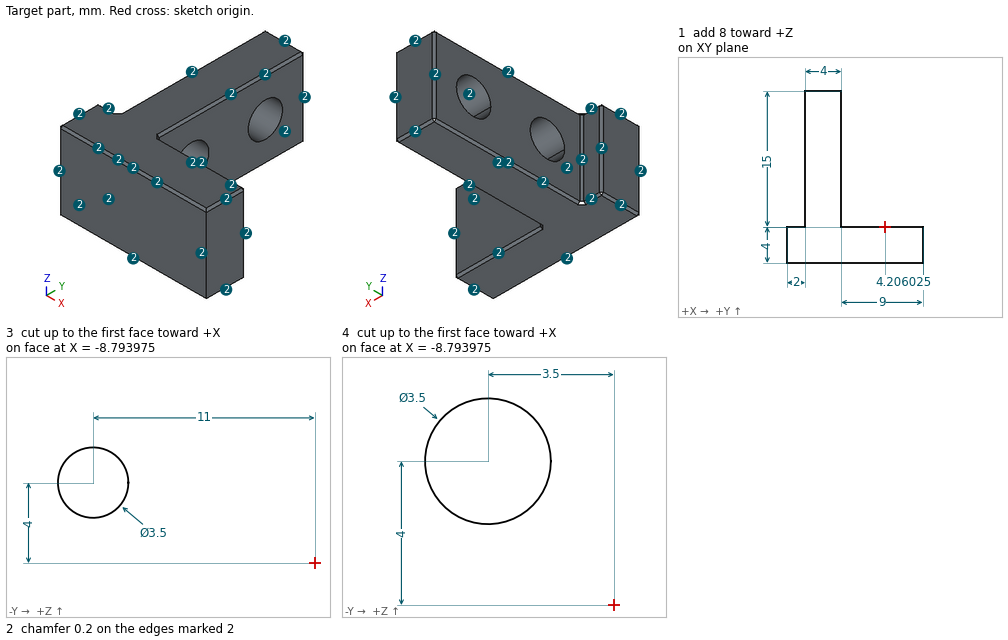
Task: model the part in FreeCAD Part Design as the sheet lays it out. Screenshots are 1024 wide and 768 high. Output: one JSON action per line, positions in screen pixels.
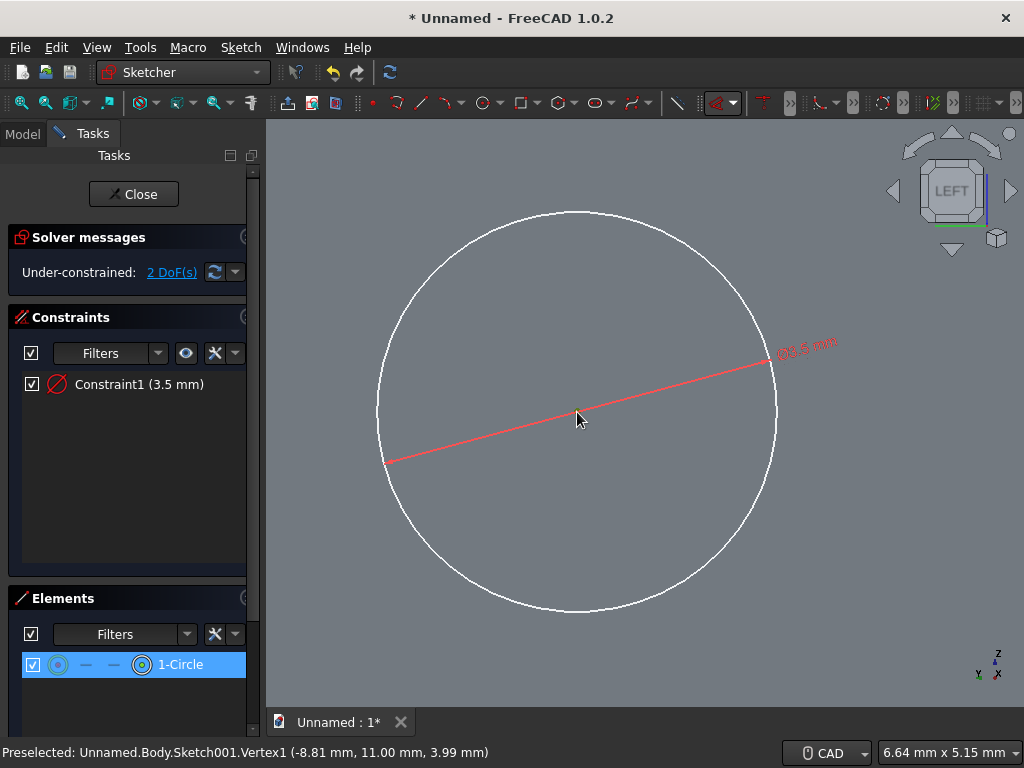
{"action": "left_click", "coordinate": [736, 104]}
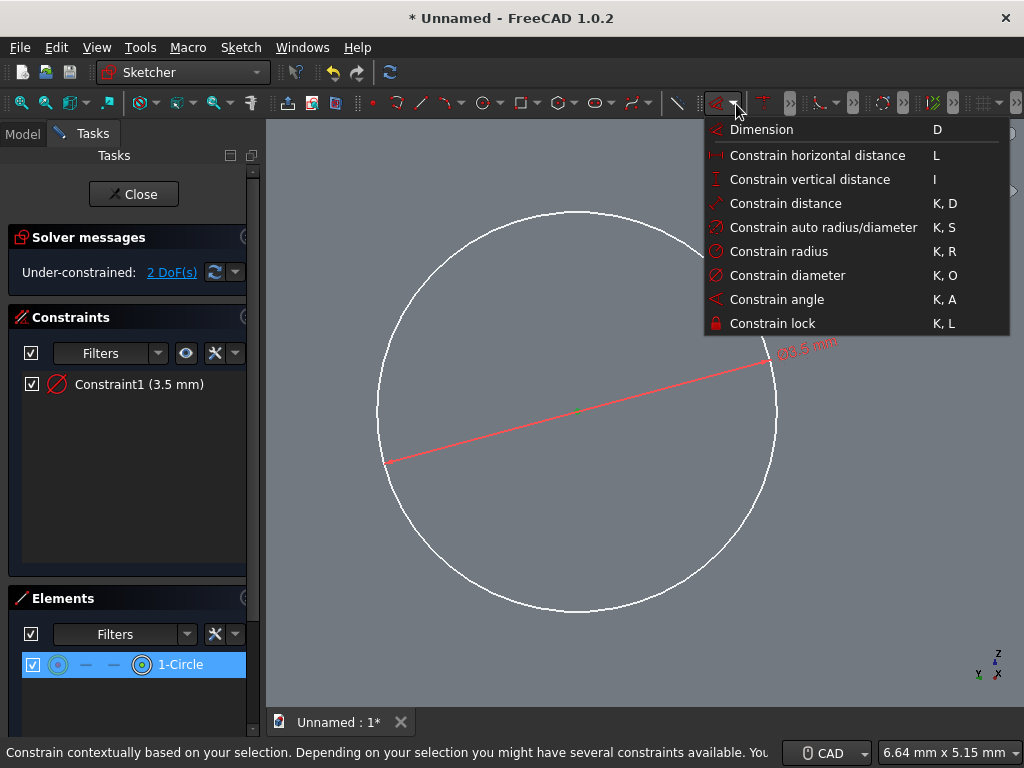
{"action": "left_click", "coordinate": [857, 179]}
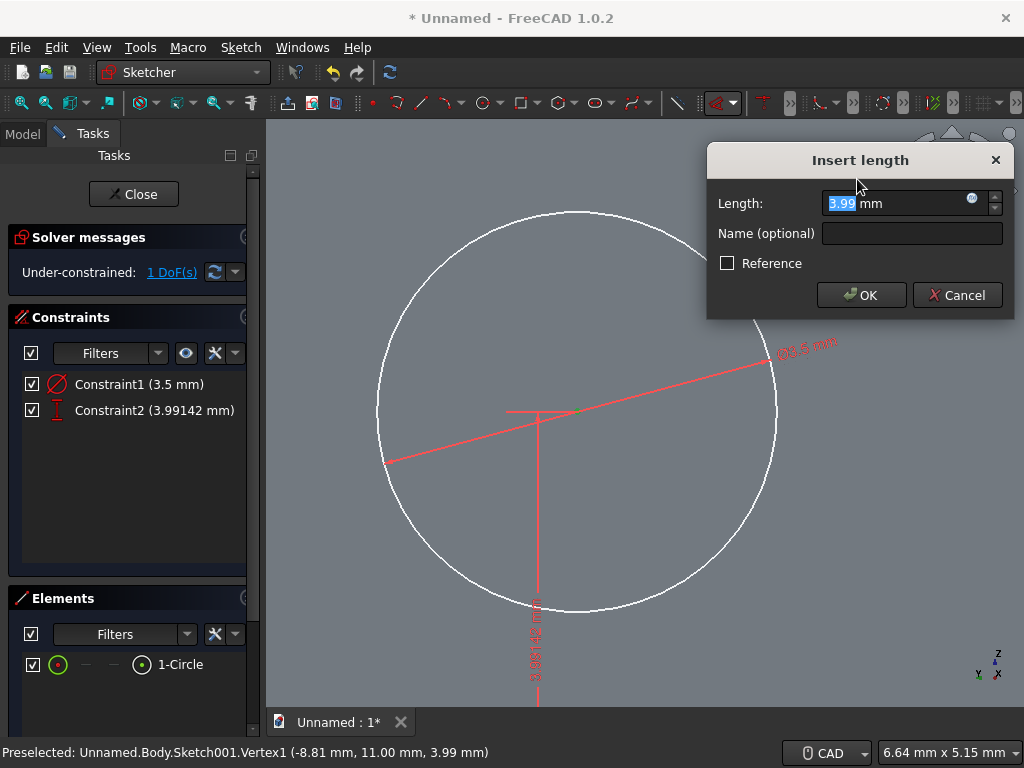
{"action": "type", "text": "4"}
{"action": "key", "text": "Return"}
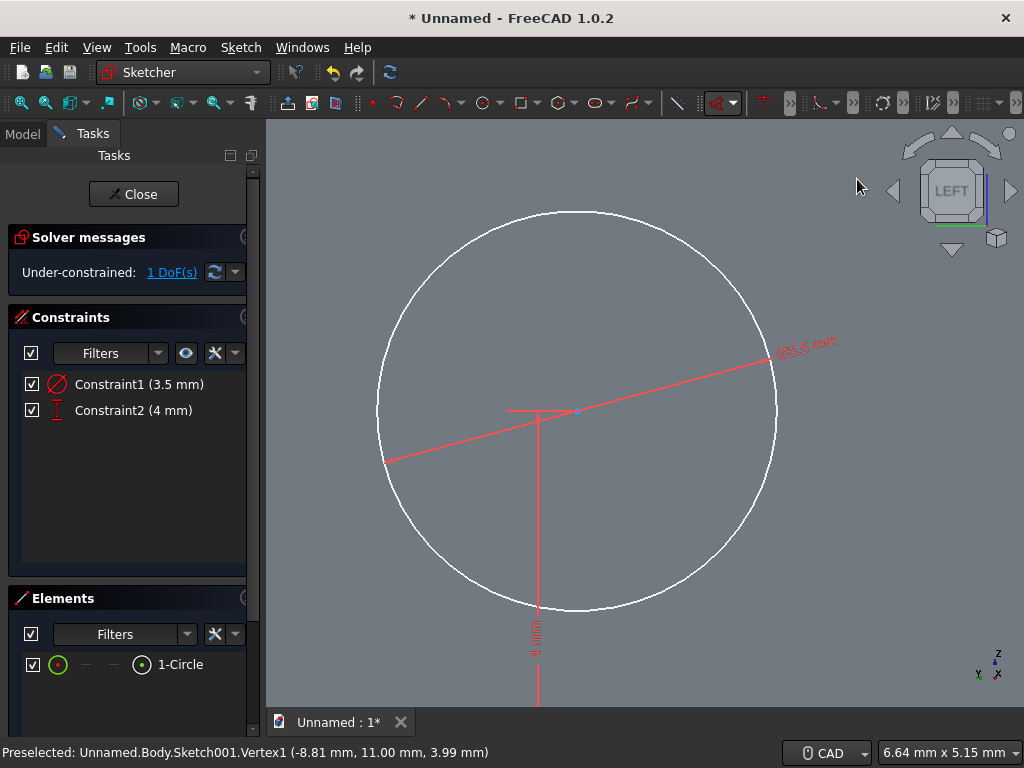
{"action": "left_click", "coordinate": [577, 411]}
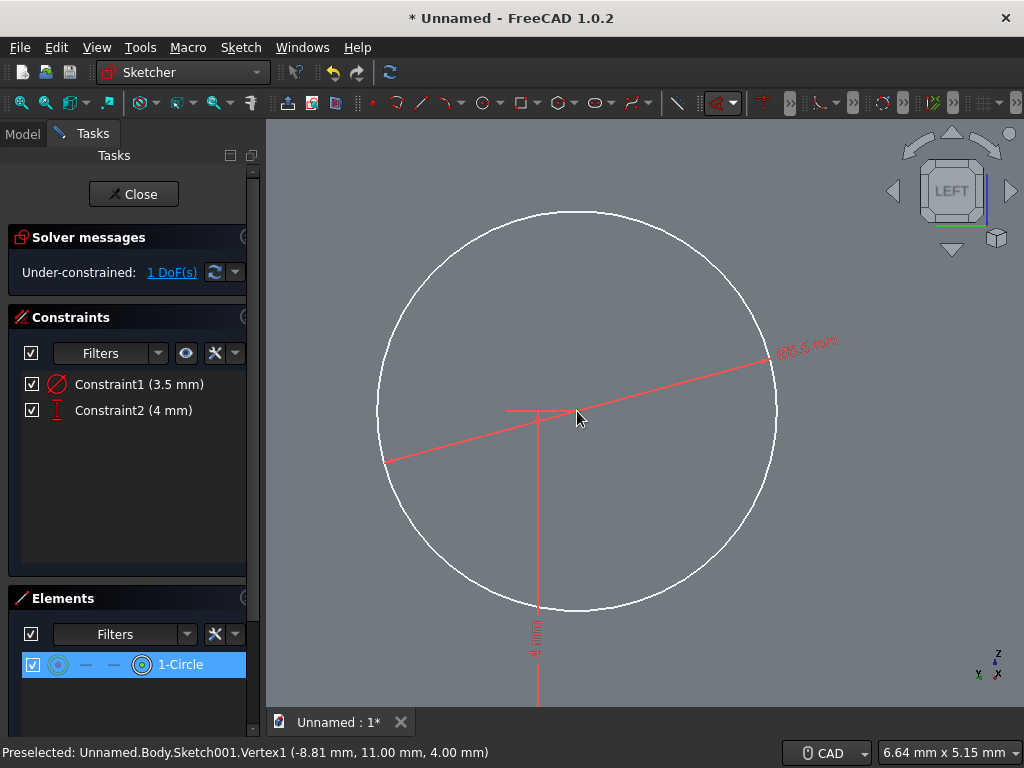
{"action": "key", "text": "l"}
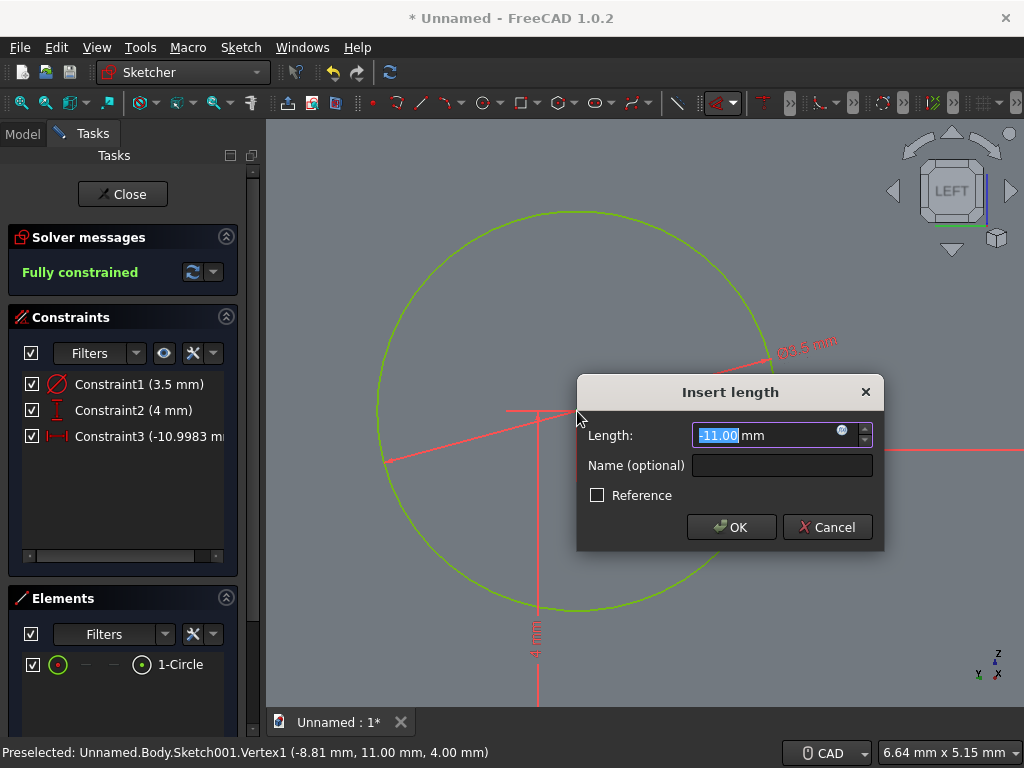
{"action": "type", "text": "-11"}
{"action": "key", "text": "Return"}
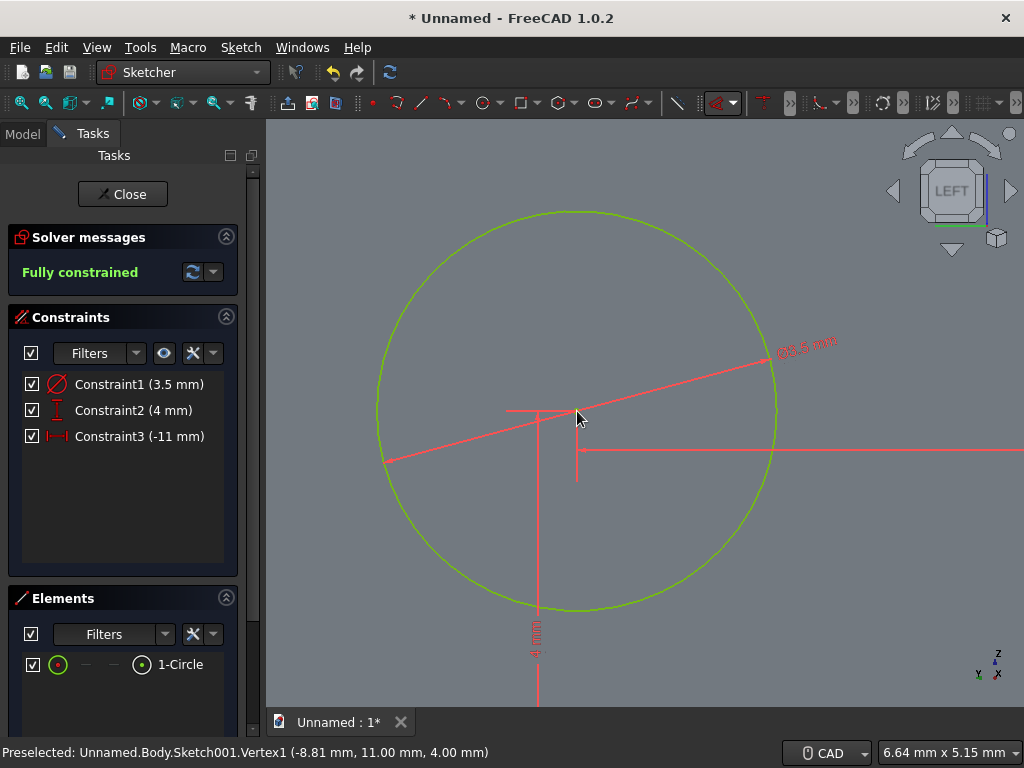
{"action": "left_click", "coordinate": [123, 194]}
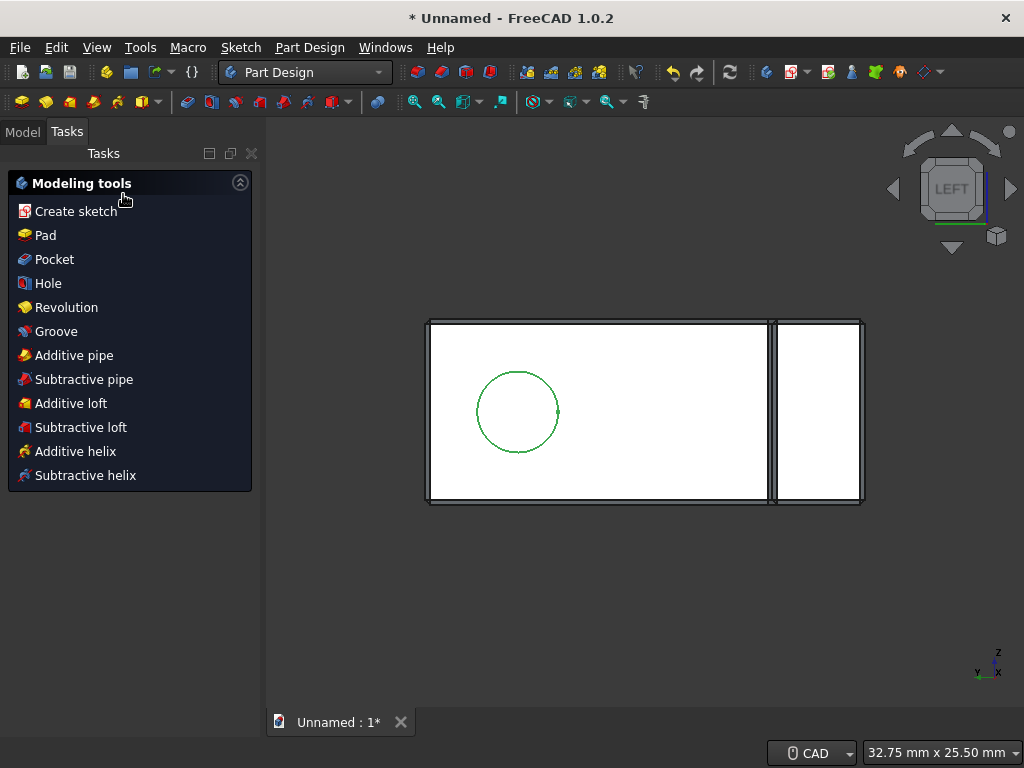
{"action": "left_click", "coordinate": [188, 102]}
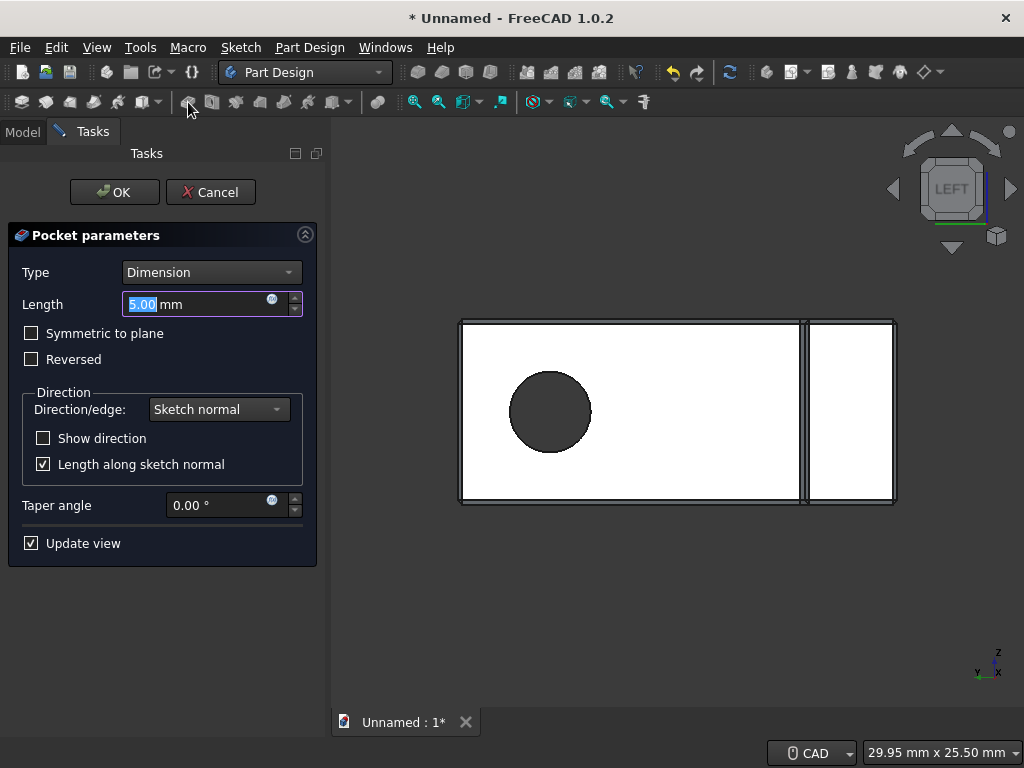
{"action": "left_click", "coordinate": [212, 272]}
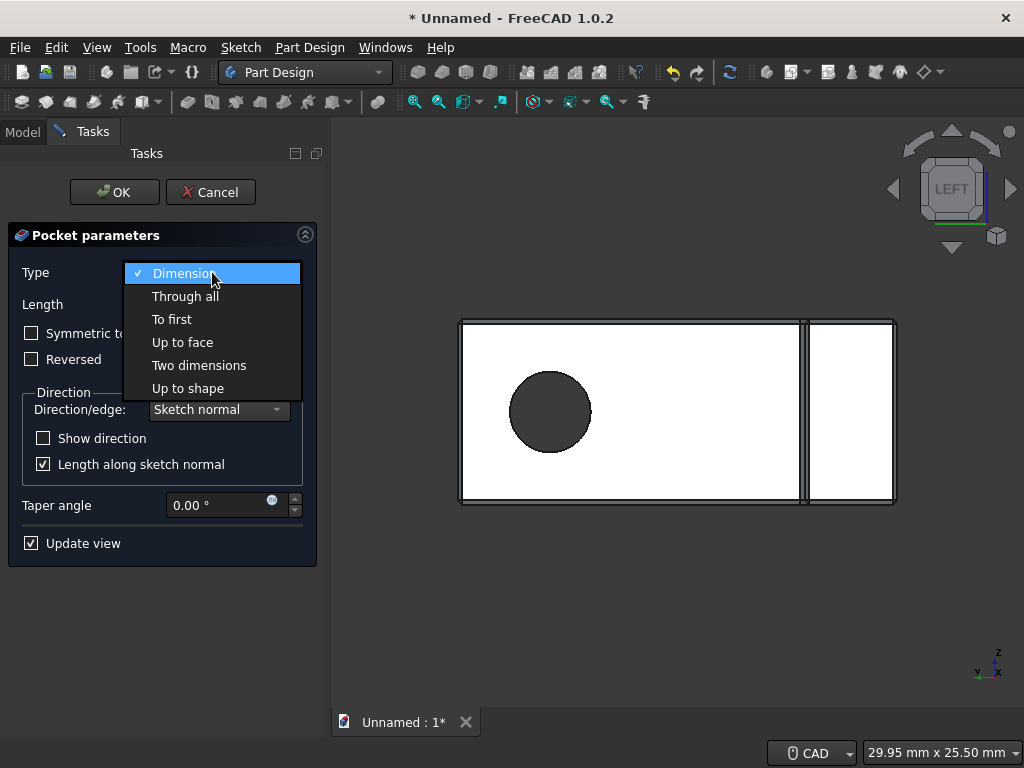
{"action": "left_click", "coordinate": [212, 320]}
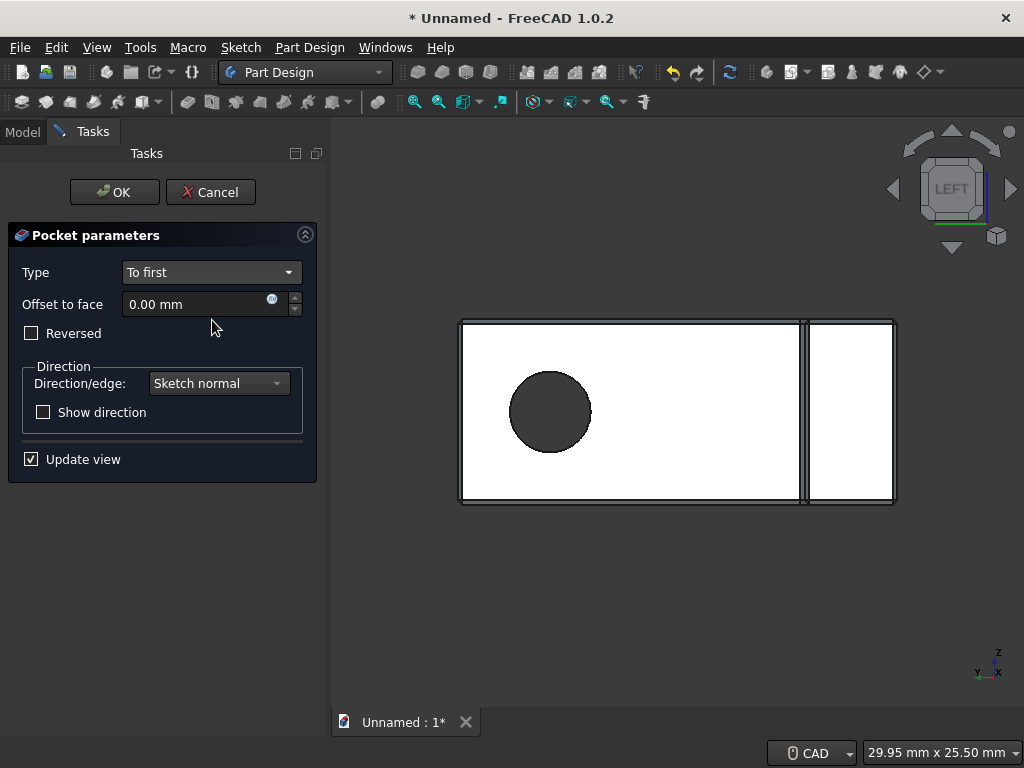
{"action": "left_click", "coordinate": [115, 192]}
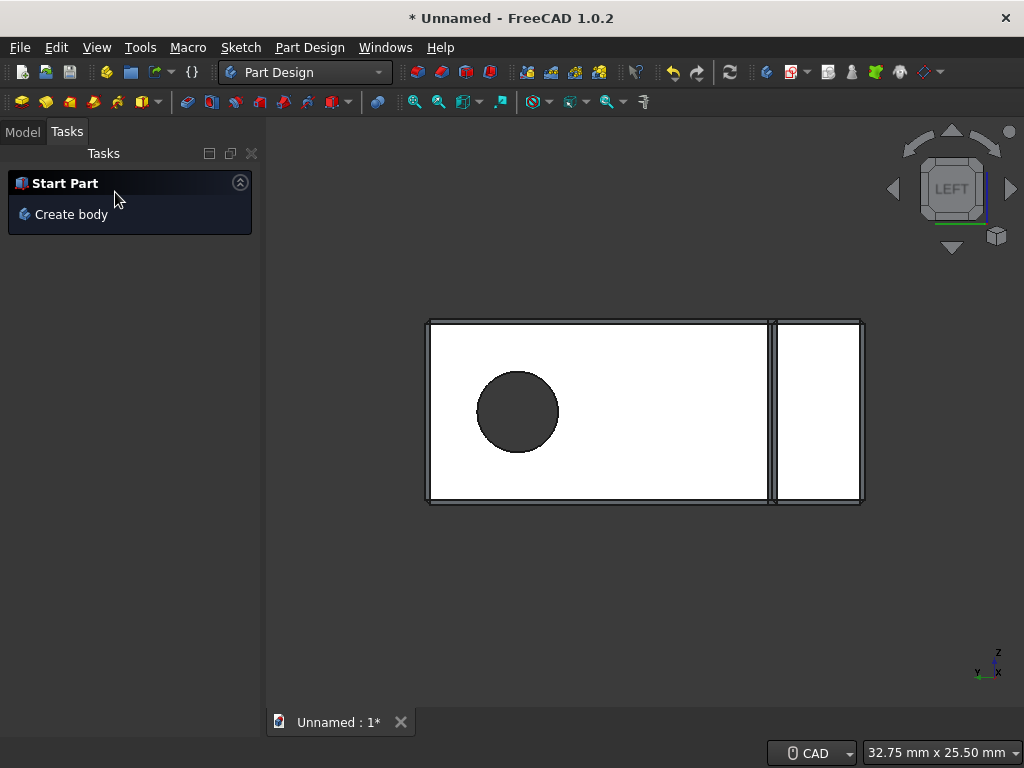
{"action": "left_click", "coordinate": [647, 411]}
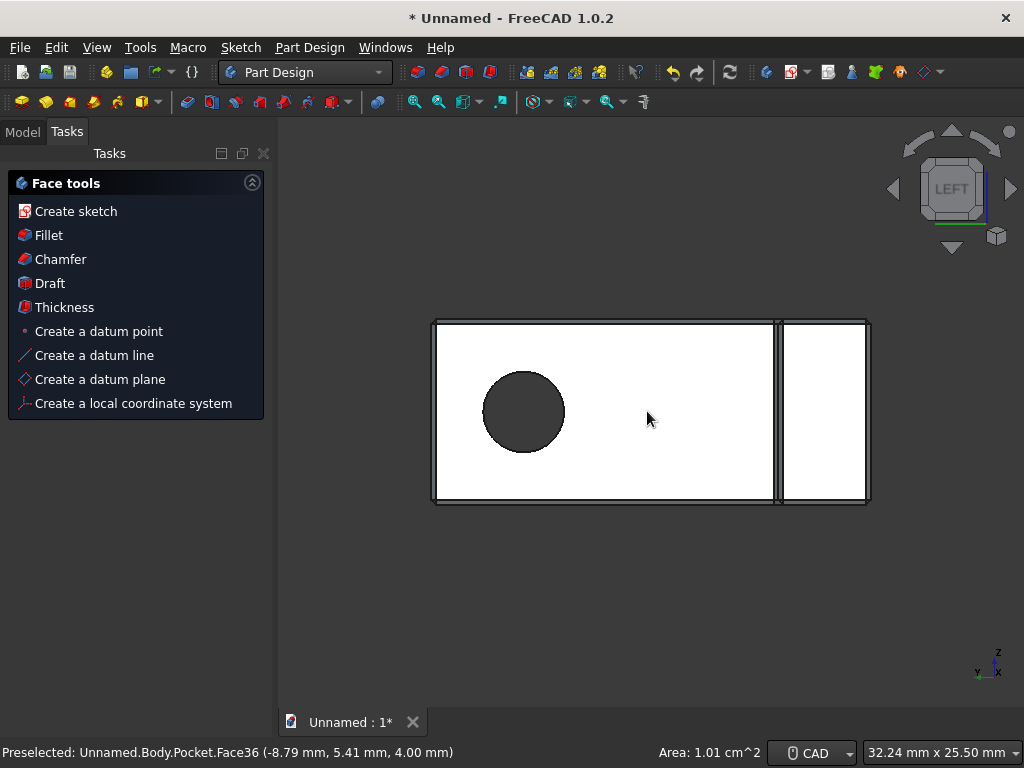
{"action": "left_click", "coordinate": [792, 72]}